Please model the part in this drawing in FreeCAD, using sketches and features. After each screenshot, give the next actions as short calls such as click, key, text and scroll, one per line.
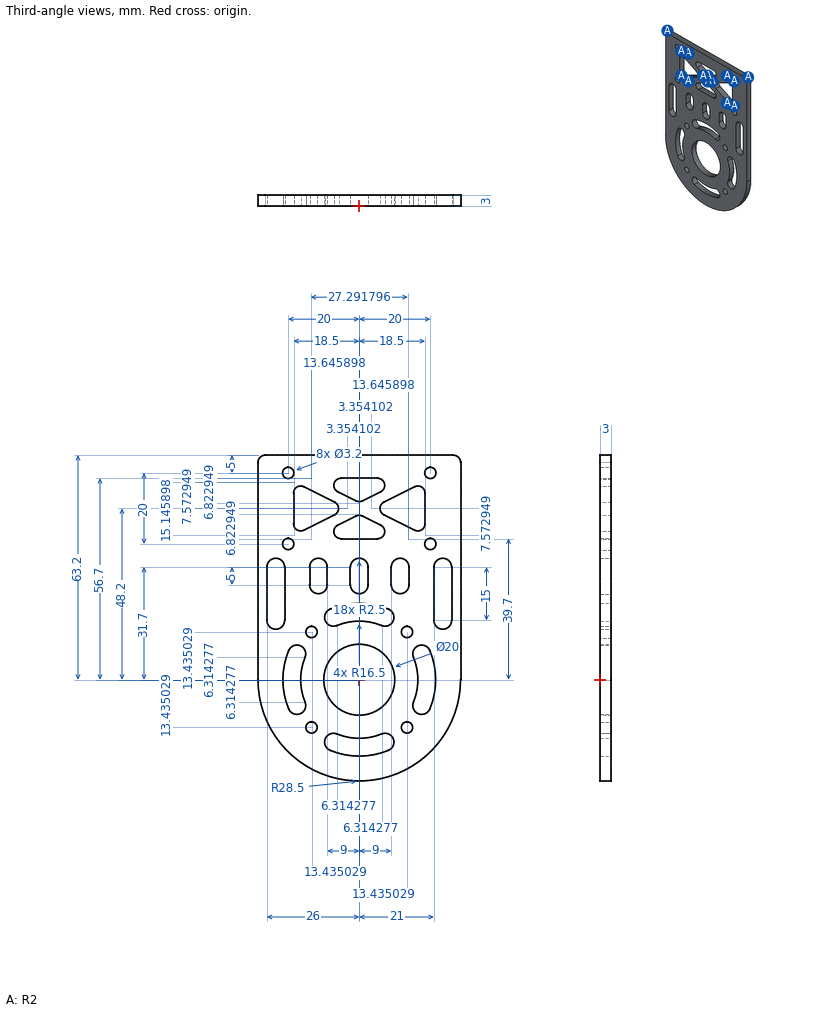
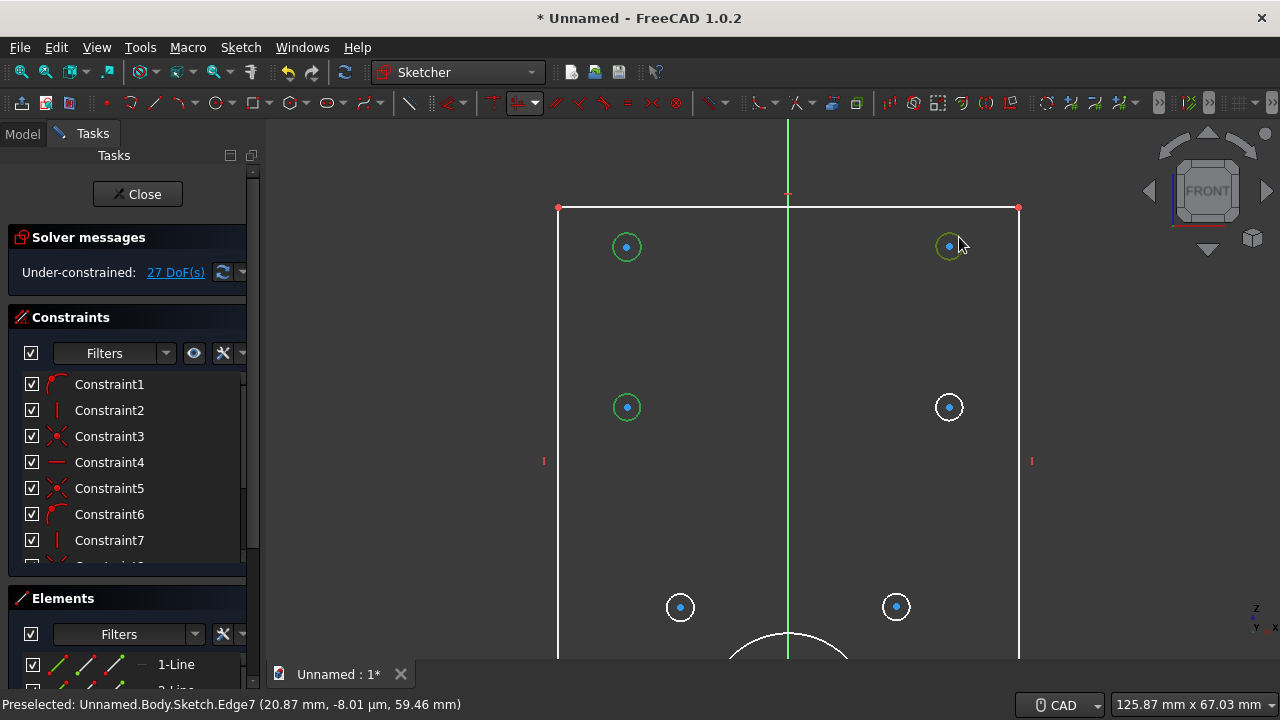
click(959, 398)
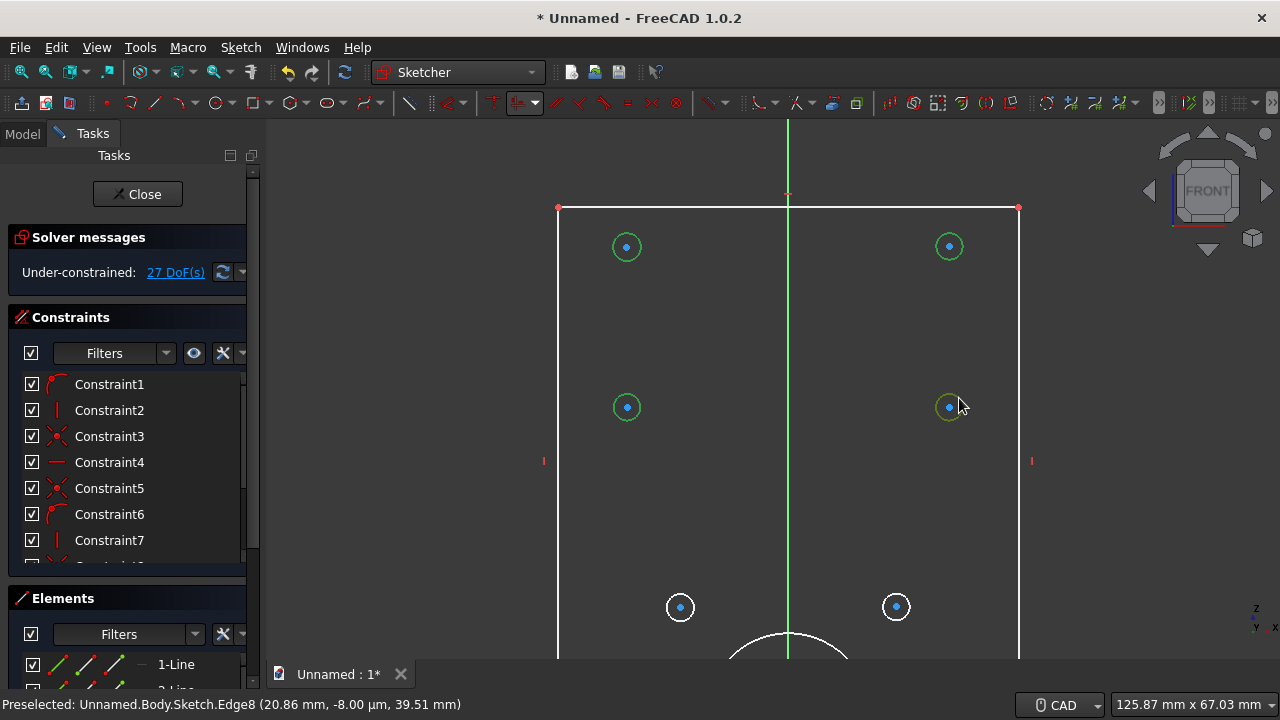
click(690, 598)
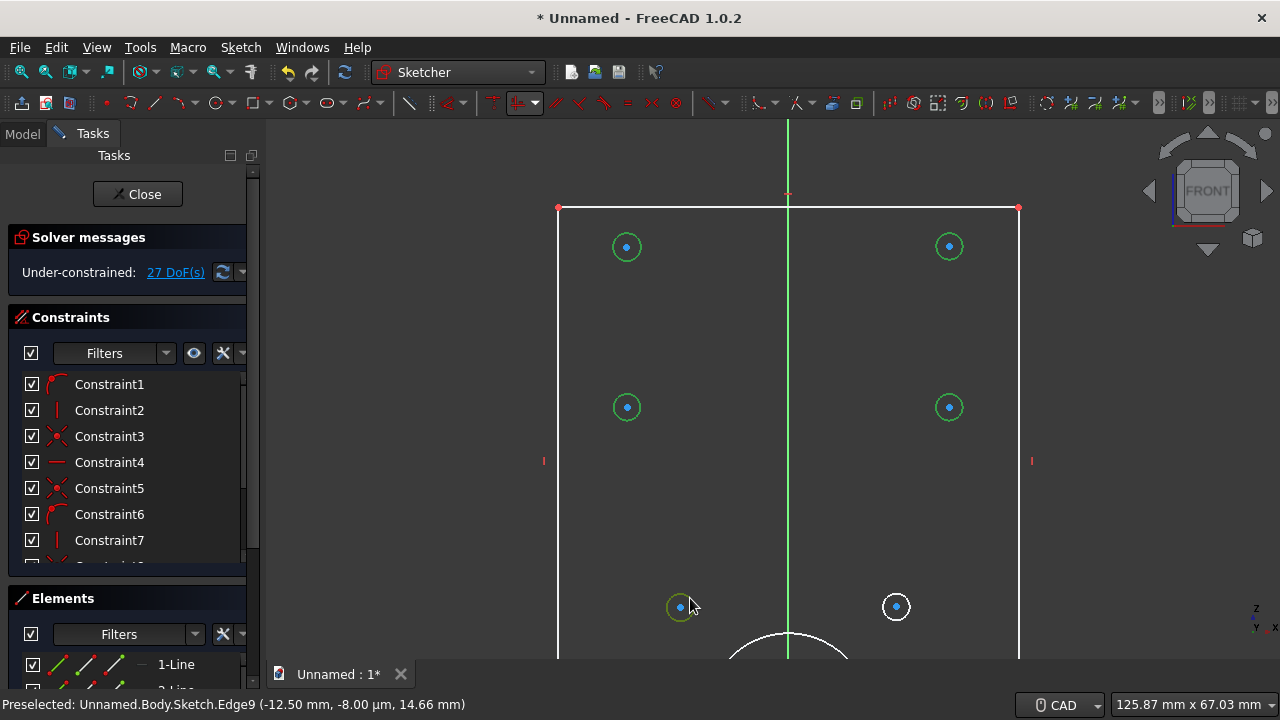
scroll(636, 238, down, 4)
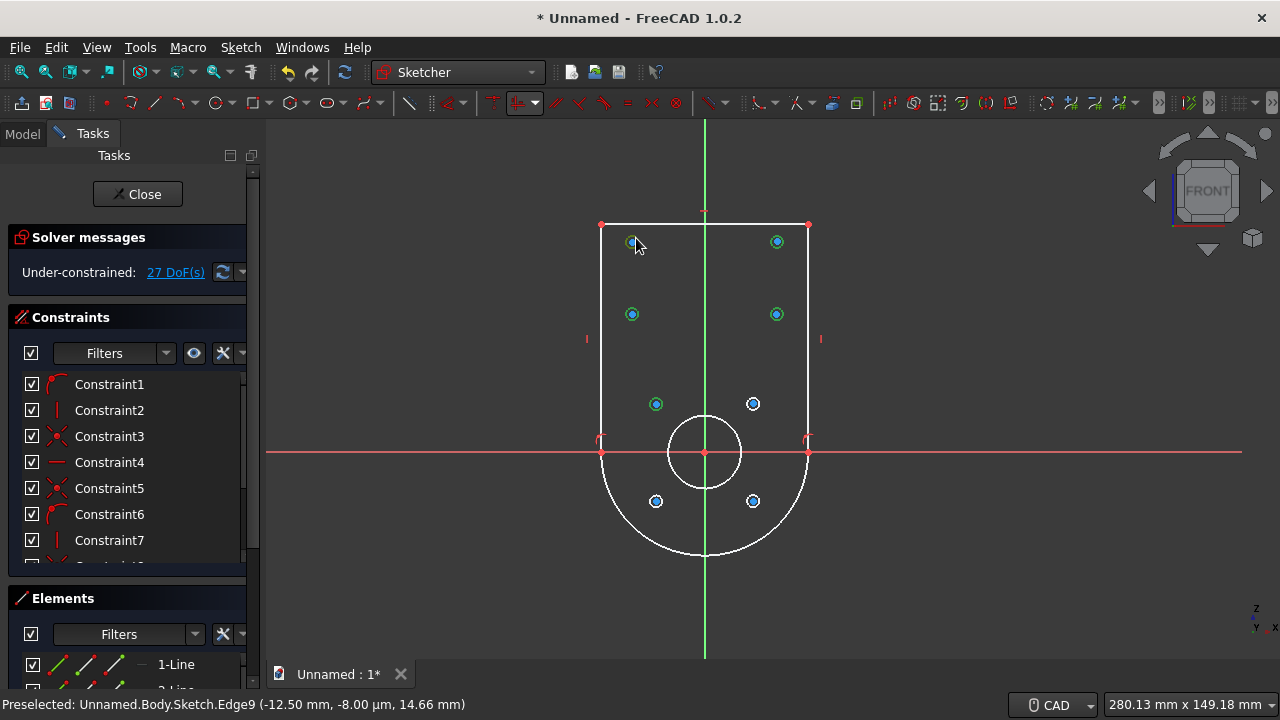
scroll(660, 497, up, 5)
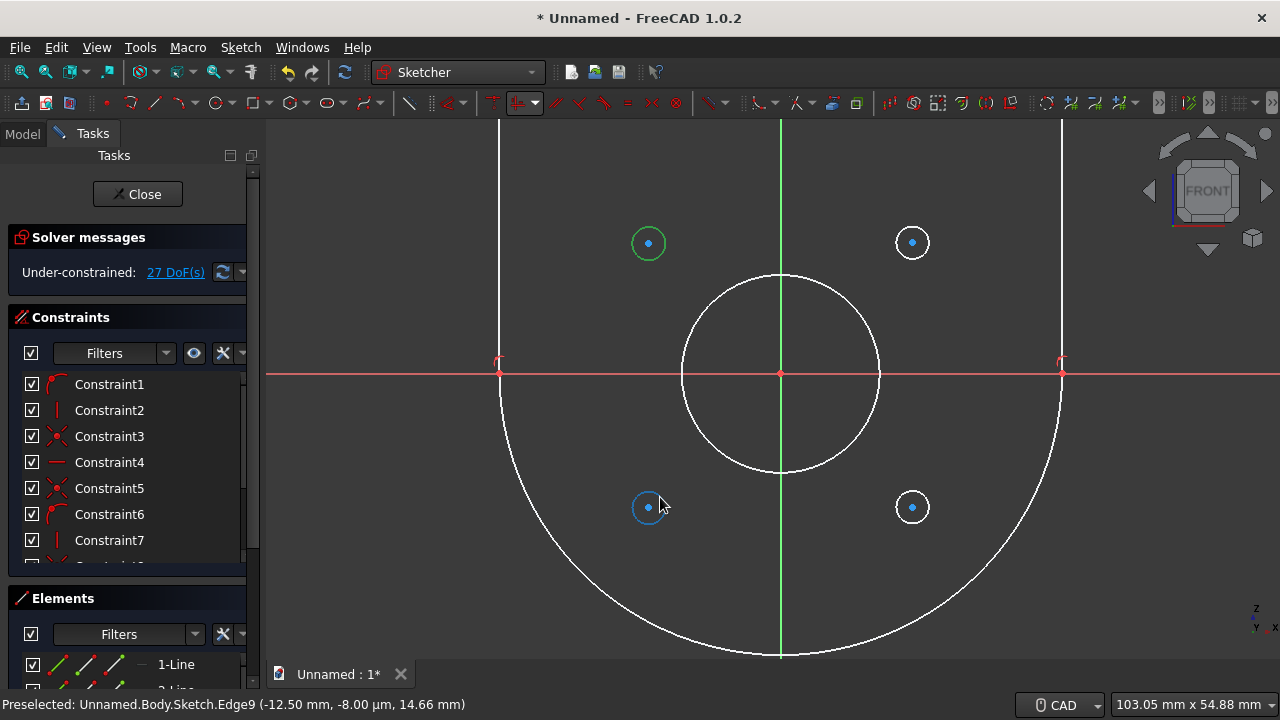
click(660, 496)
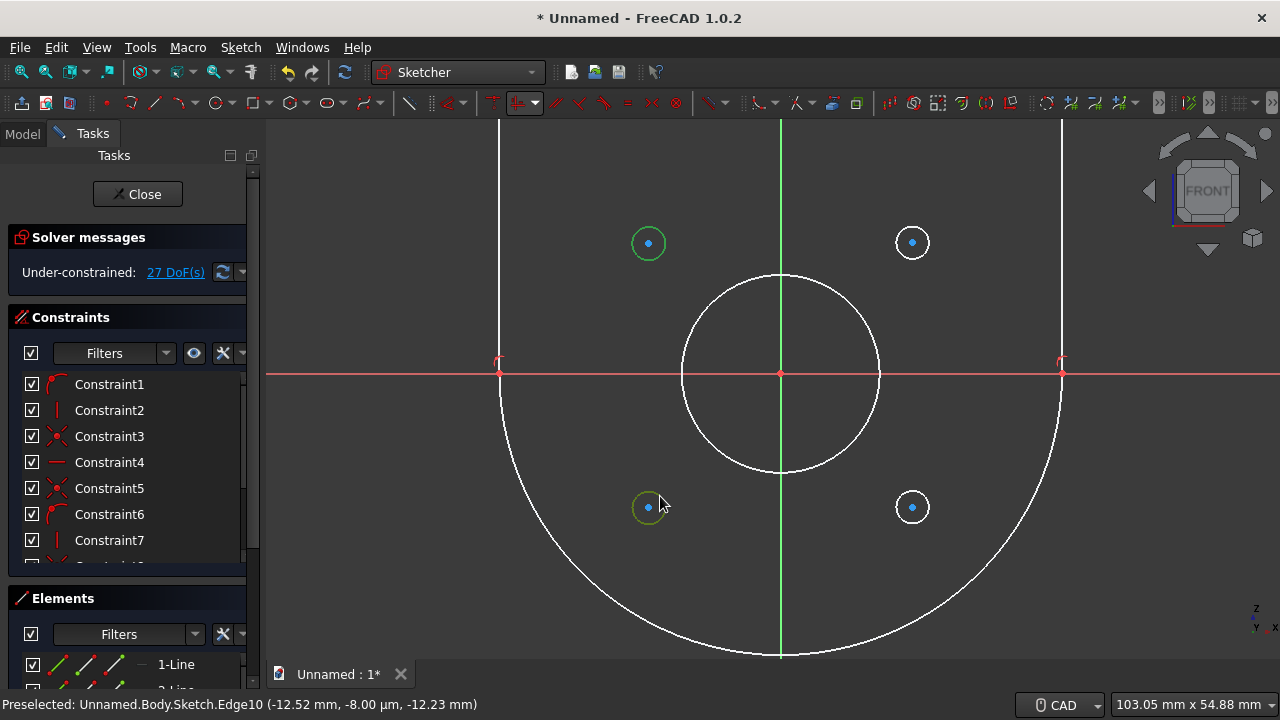
click(924, 231)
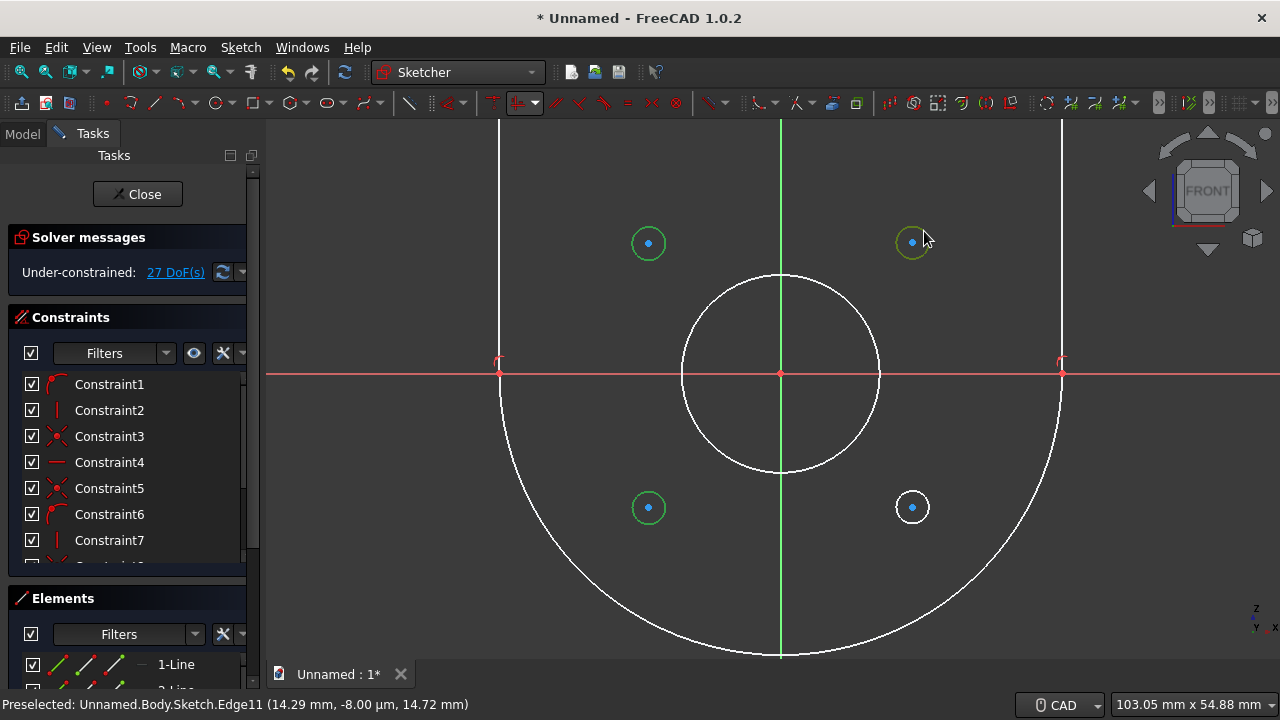
click(924, 496)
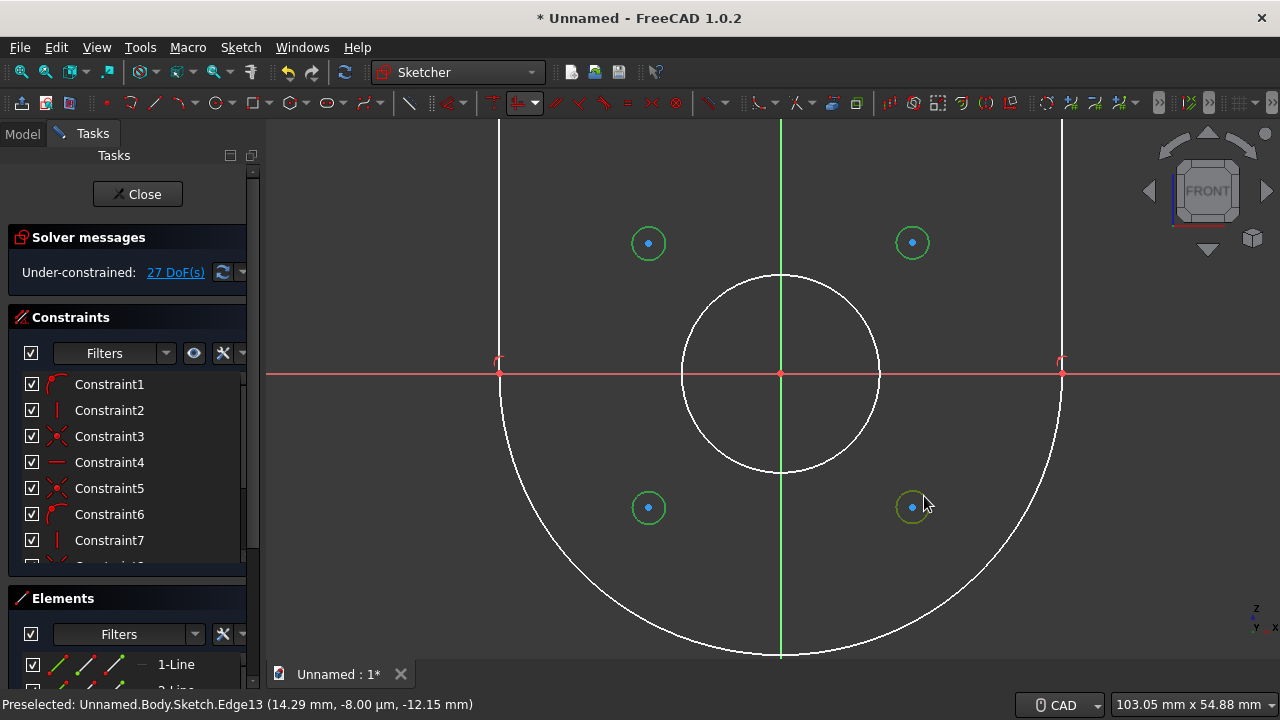
click(628, 104)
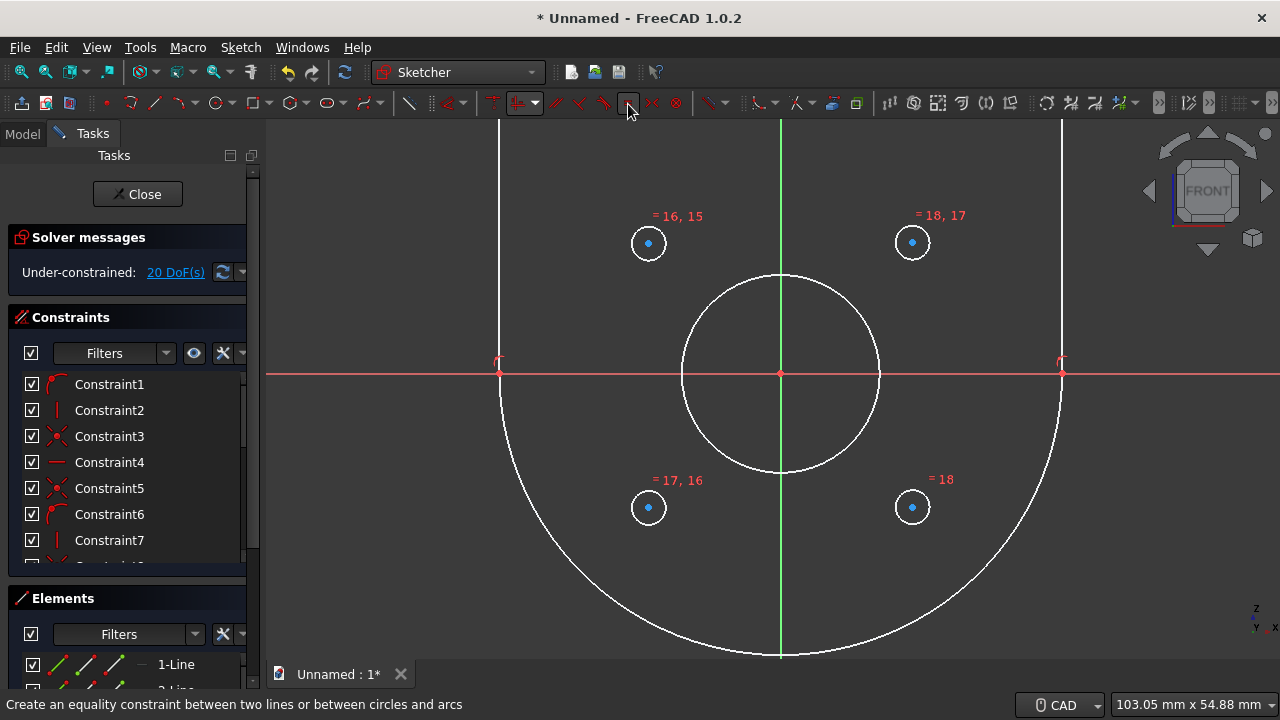
scroll(660, 497, down, 5)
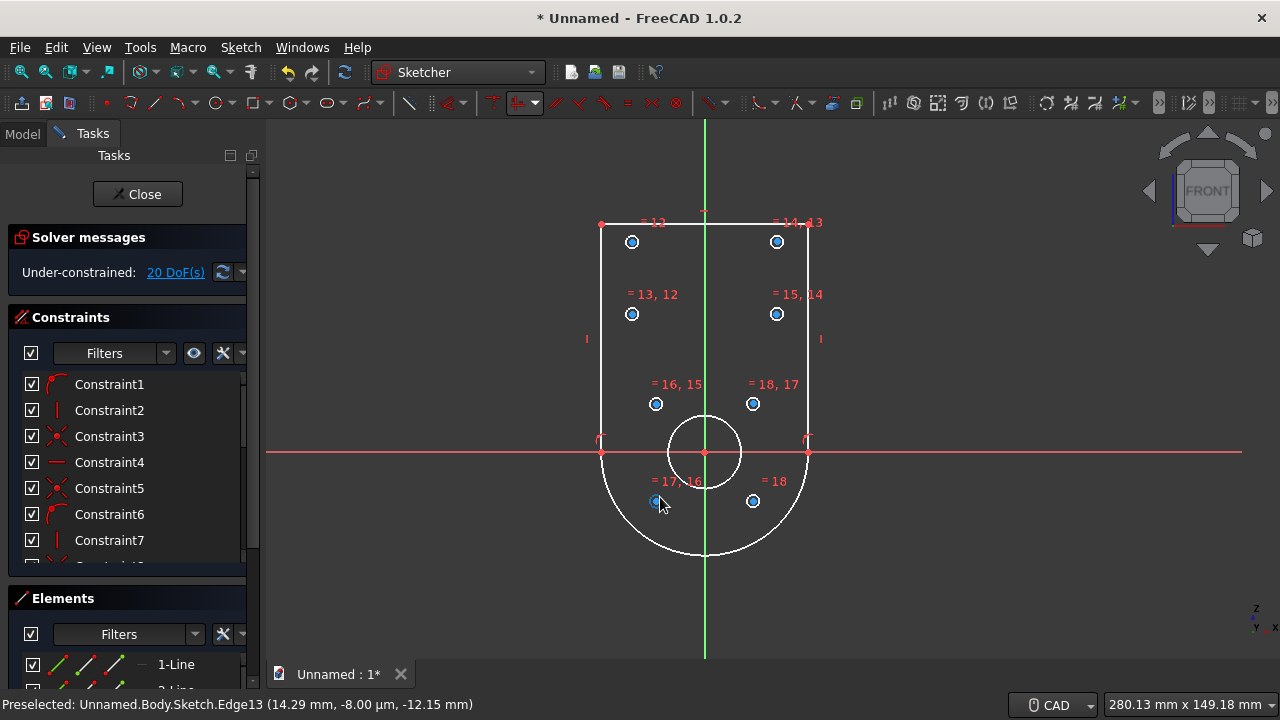
click(632, 242)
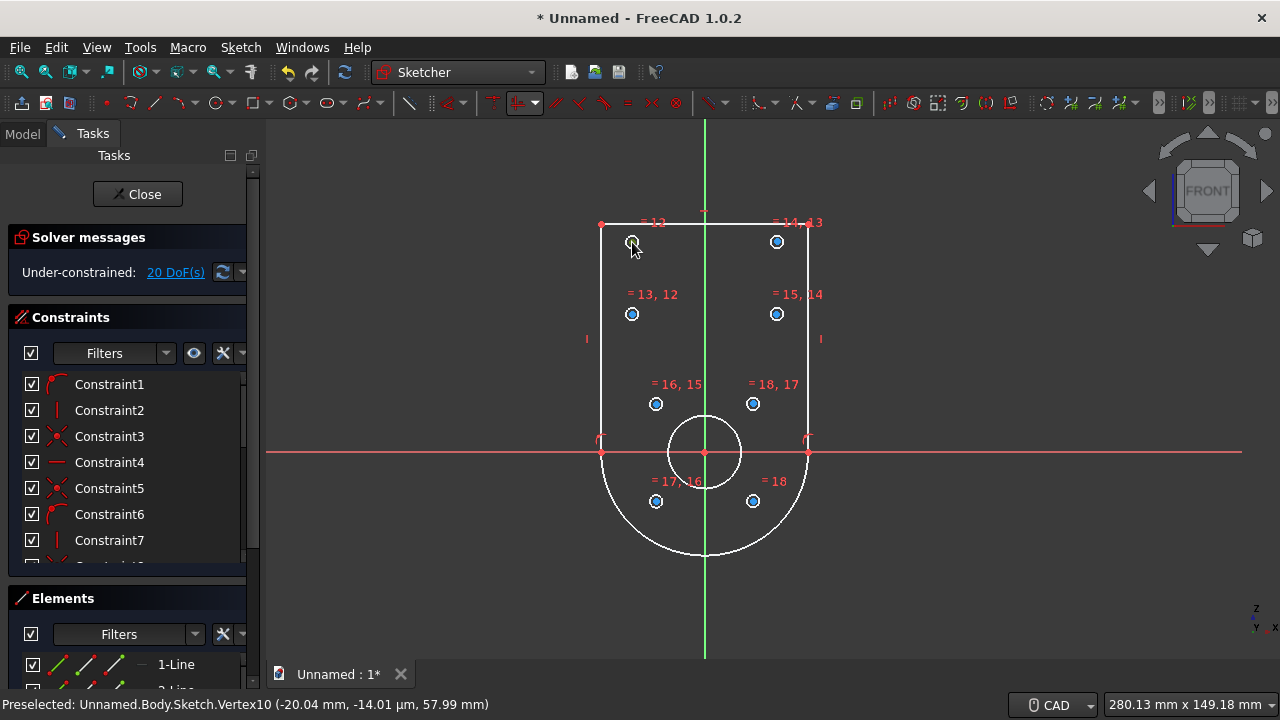
click(632, 314)